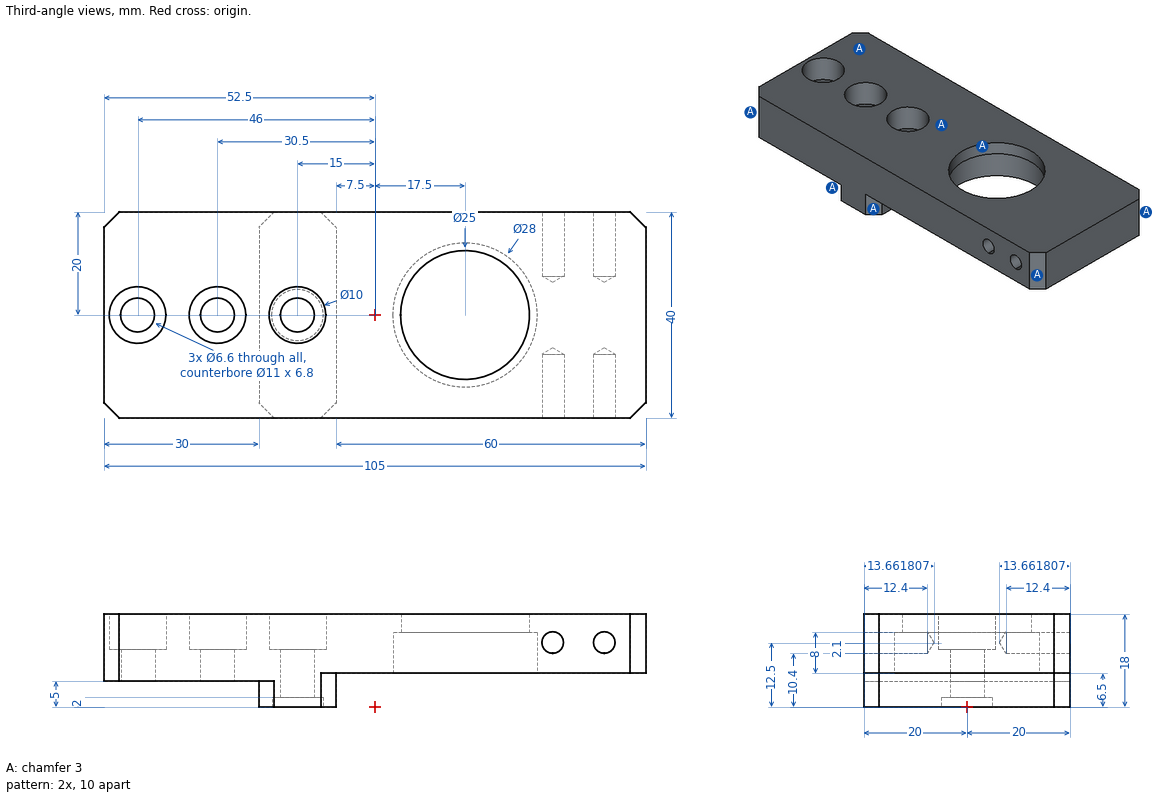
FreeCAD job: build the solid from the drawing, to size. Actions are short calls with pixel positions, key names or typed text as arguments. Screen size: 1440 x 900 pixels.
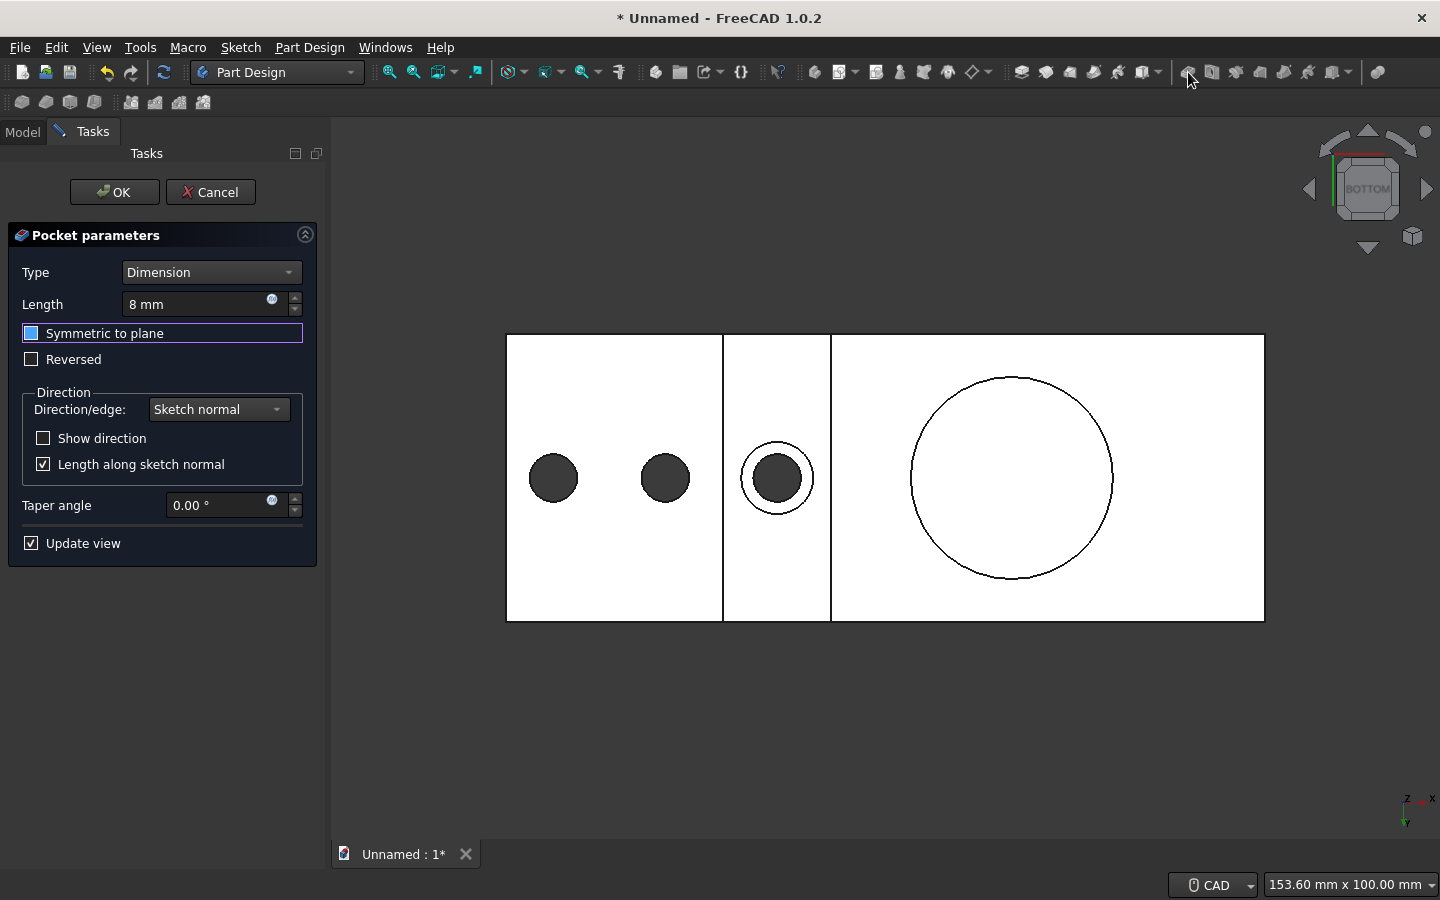
click(115, 192)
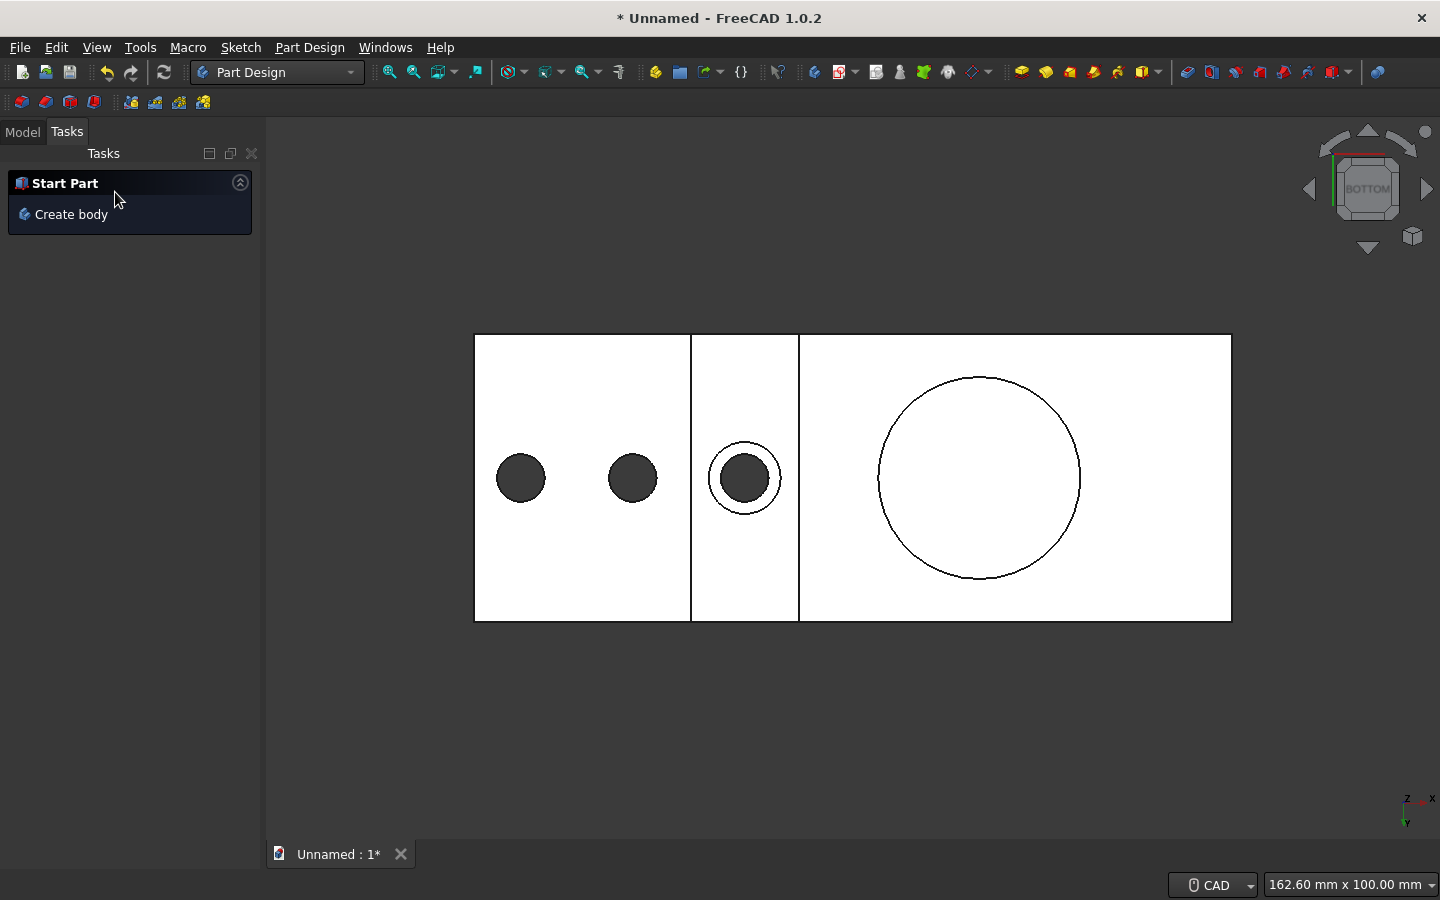
click(979, 477)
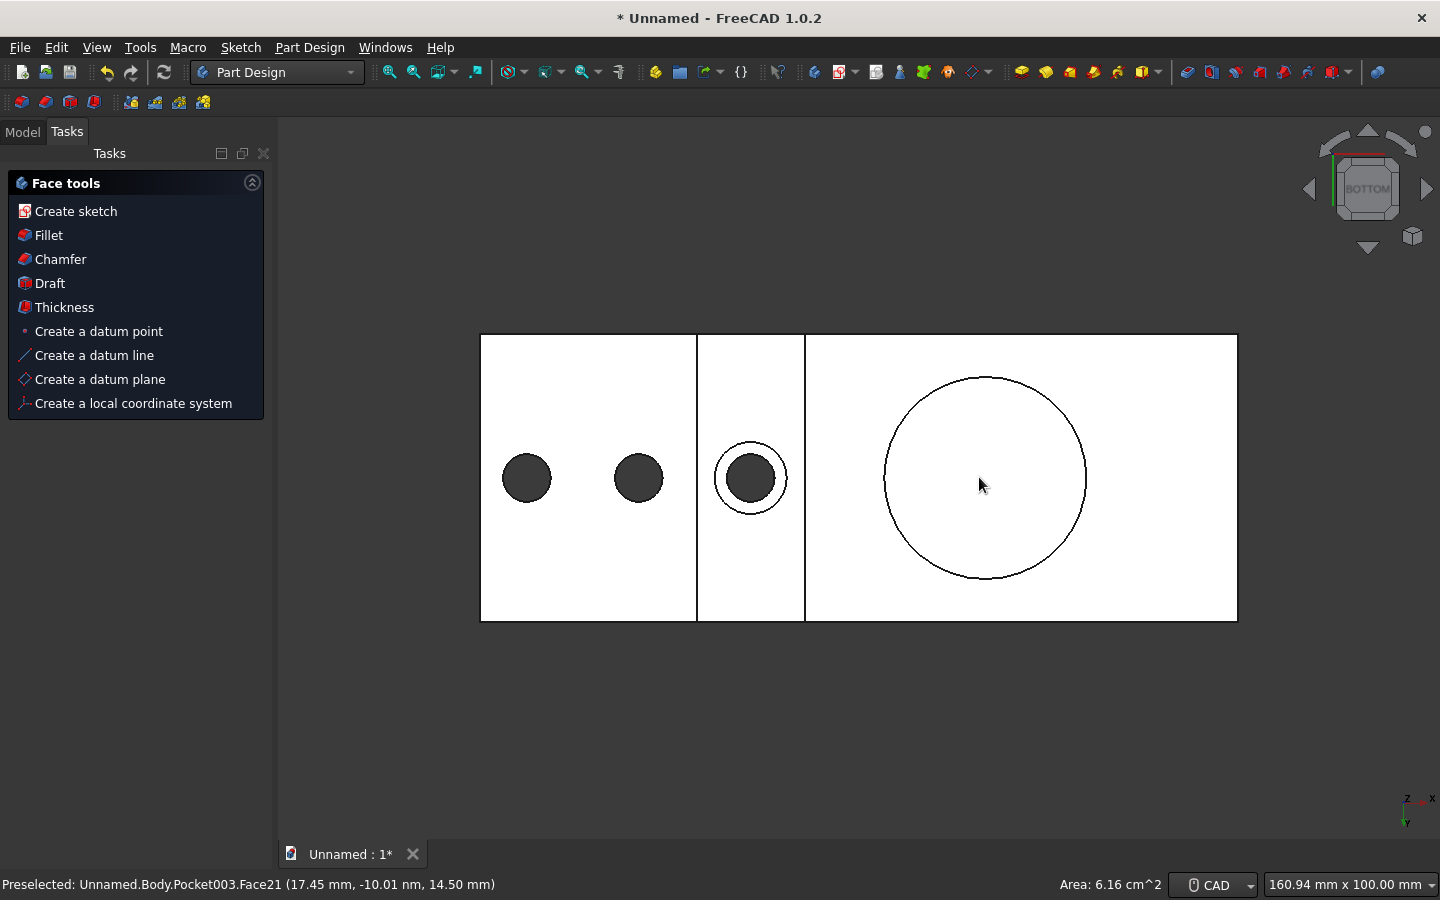
click(840, 72)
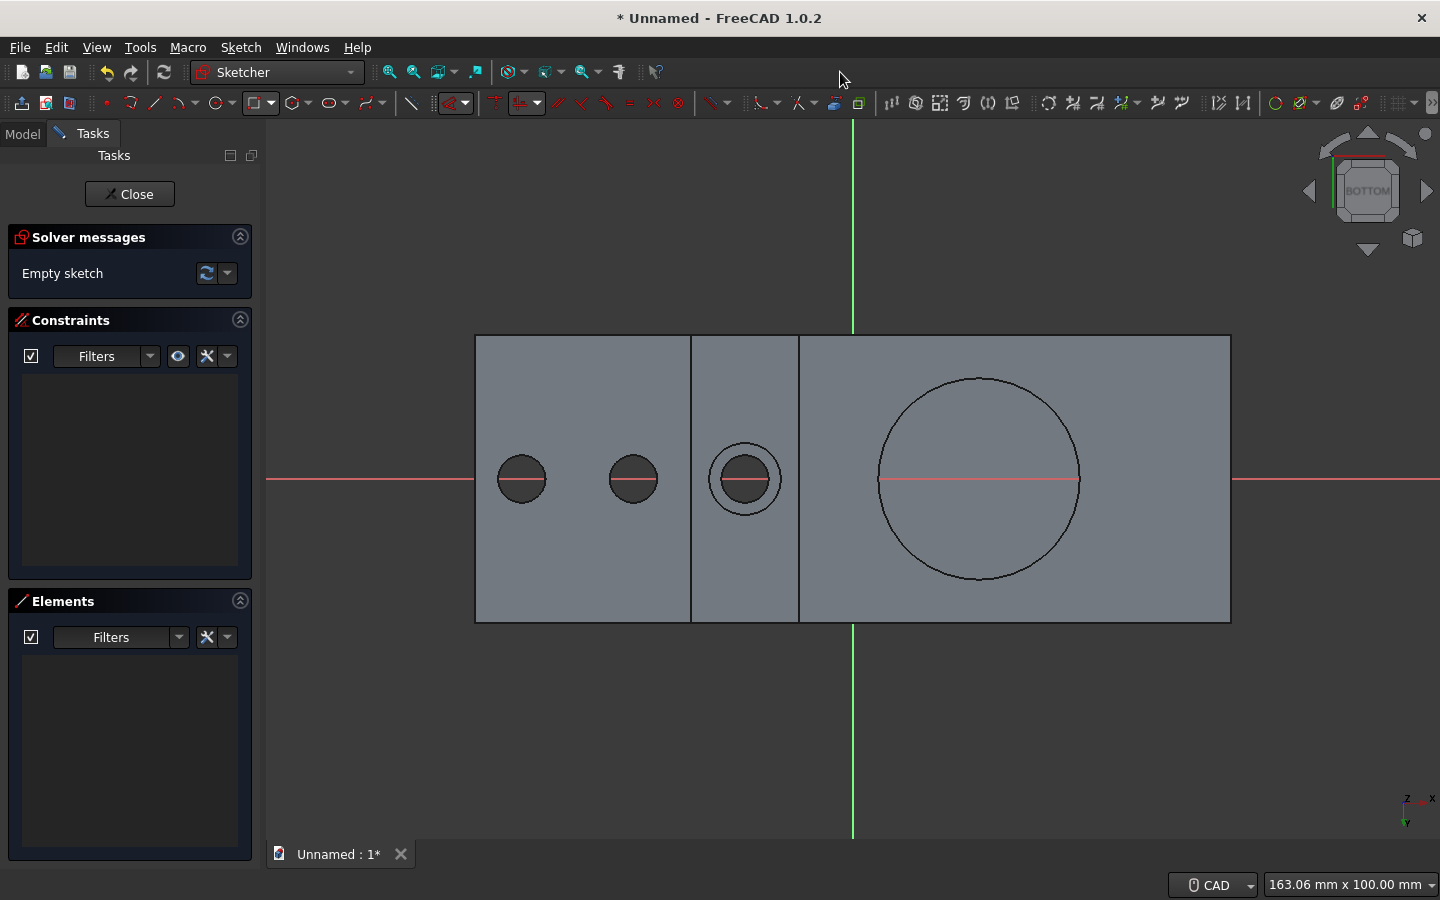
scroll(1064, 479, up, 5)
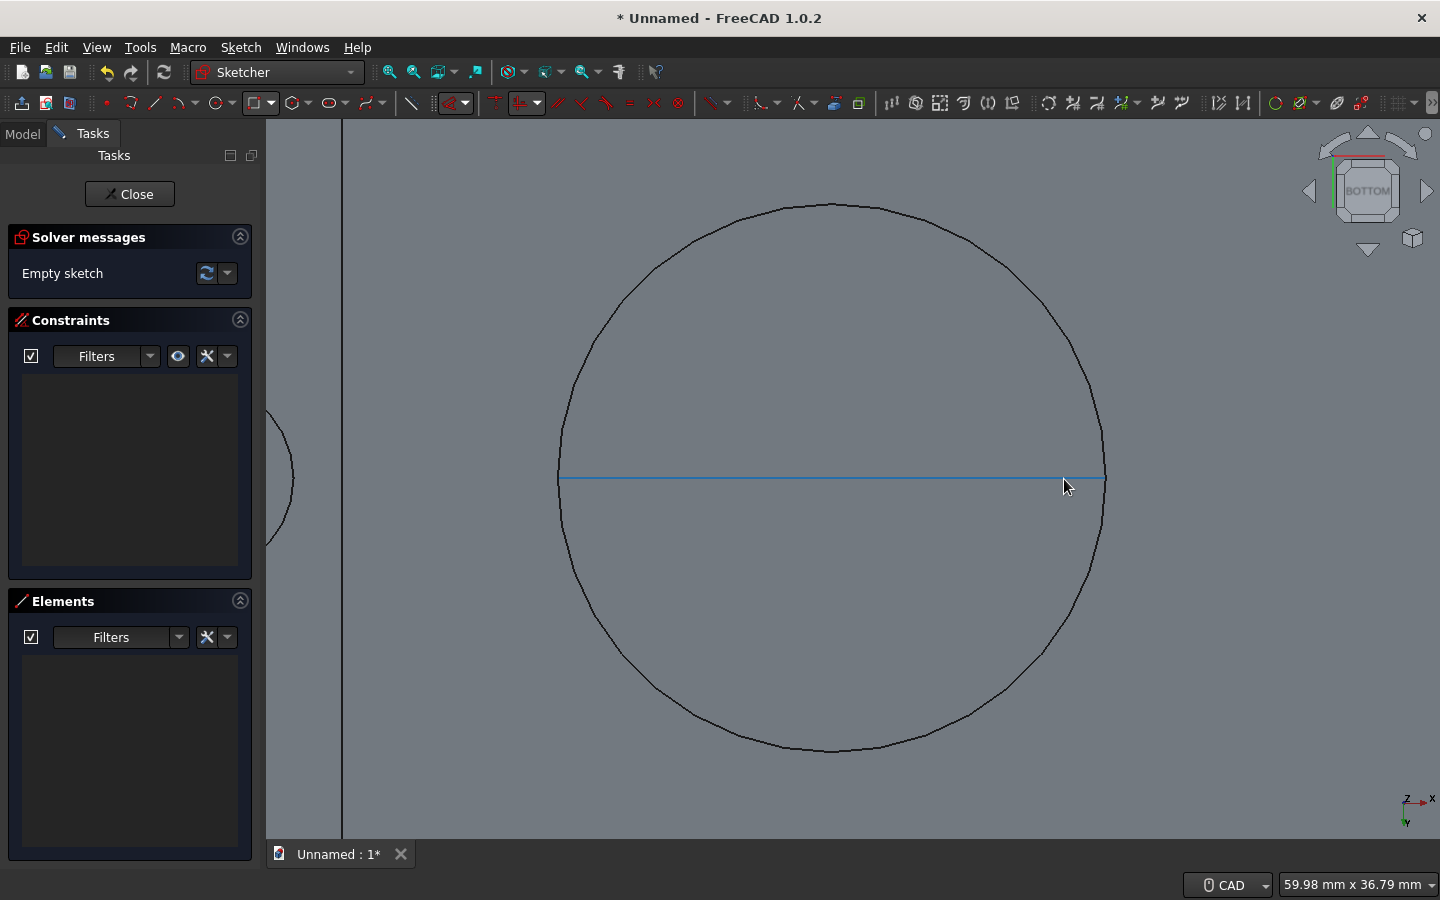
click(216, 104)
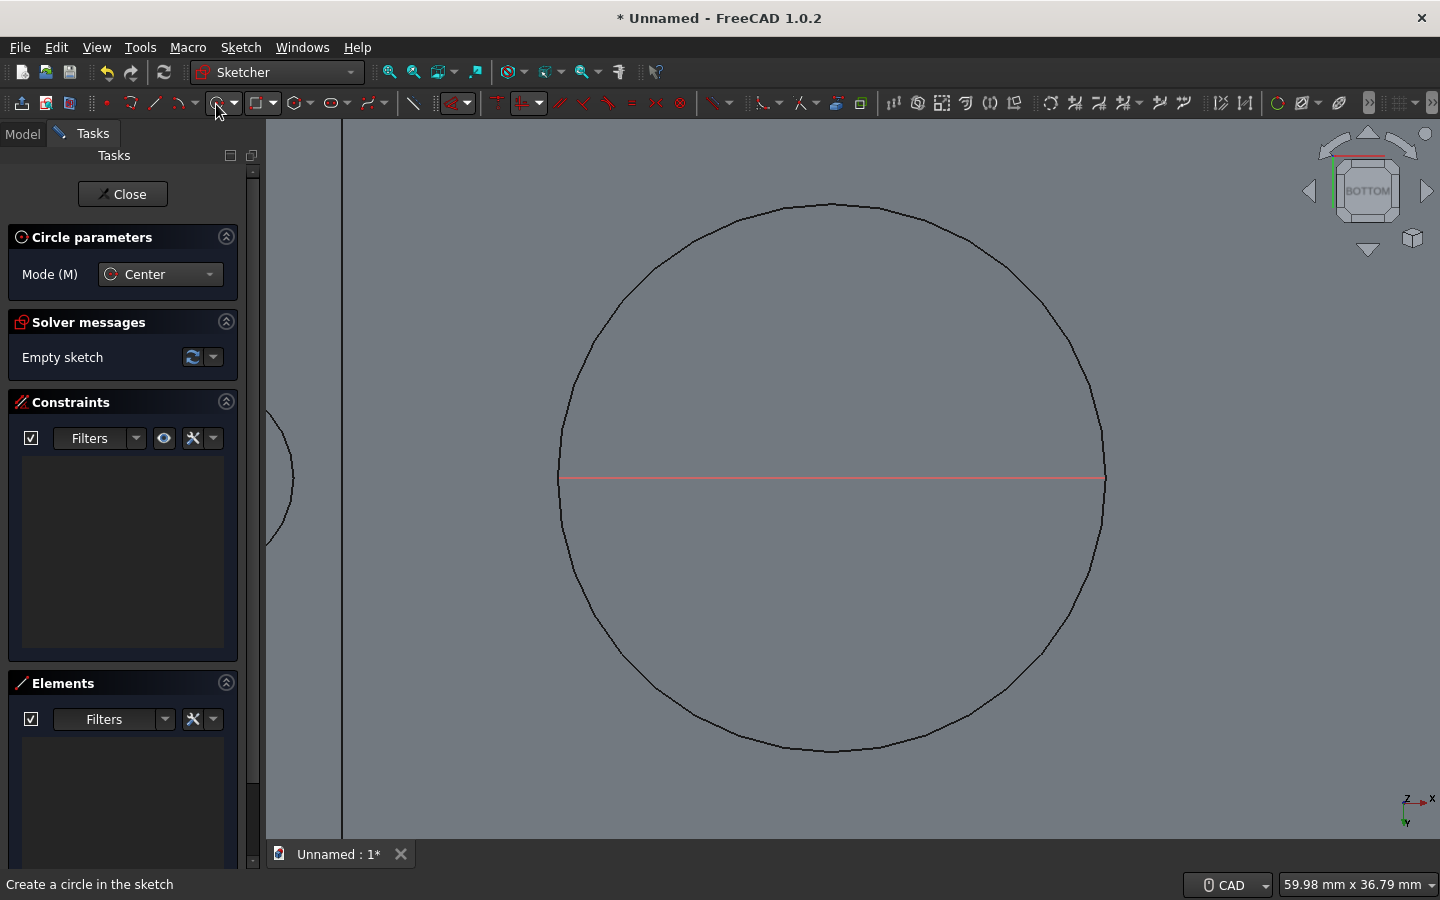
click(832, 478)
click(1005, 305)
key(Escape)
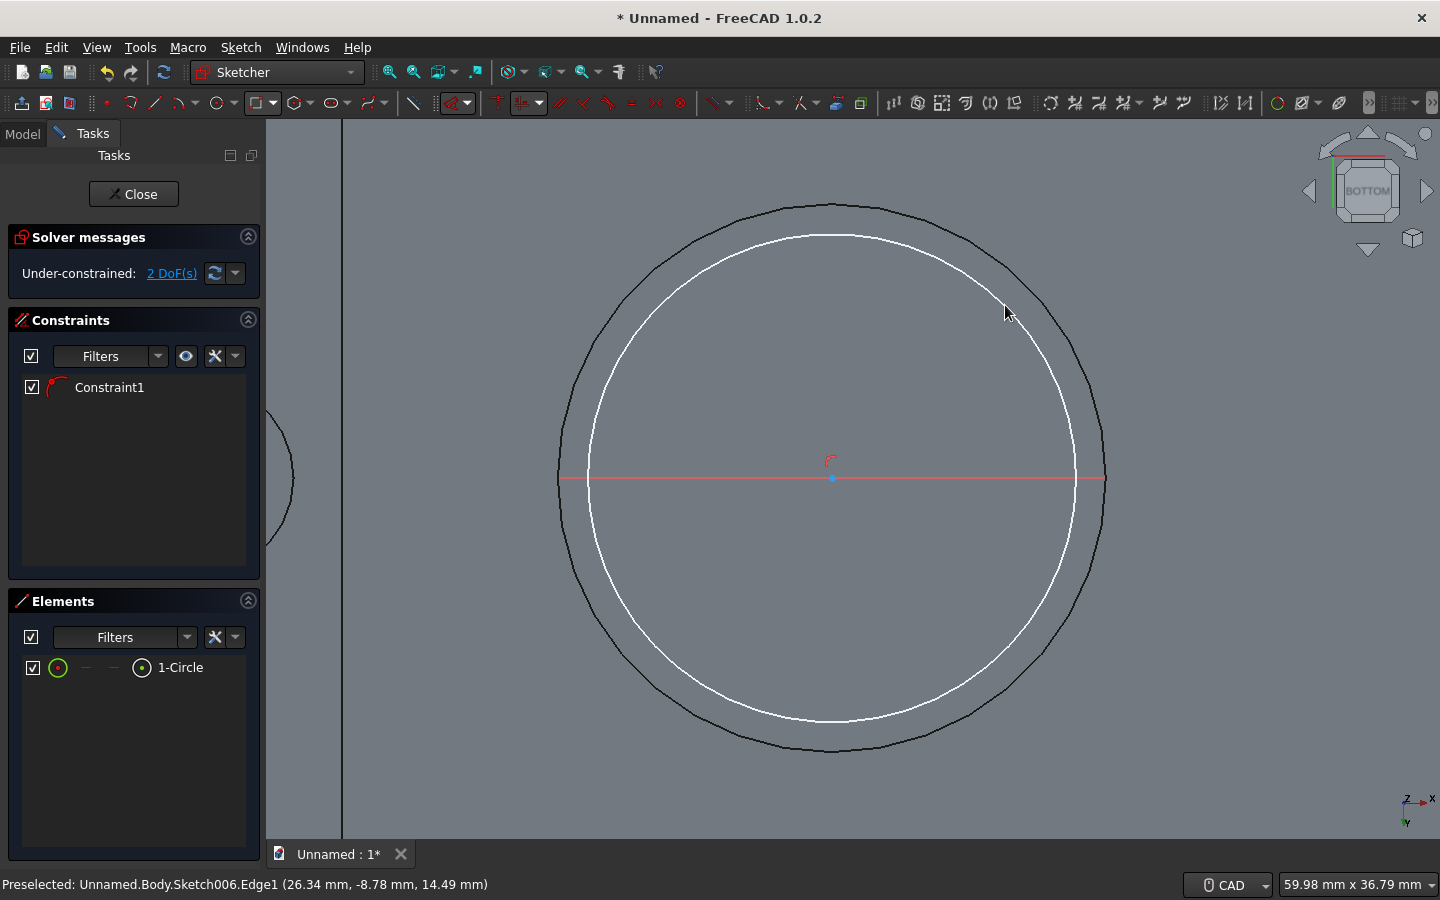
click(1004, 305)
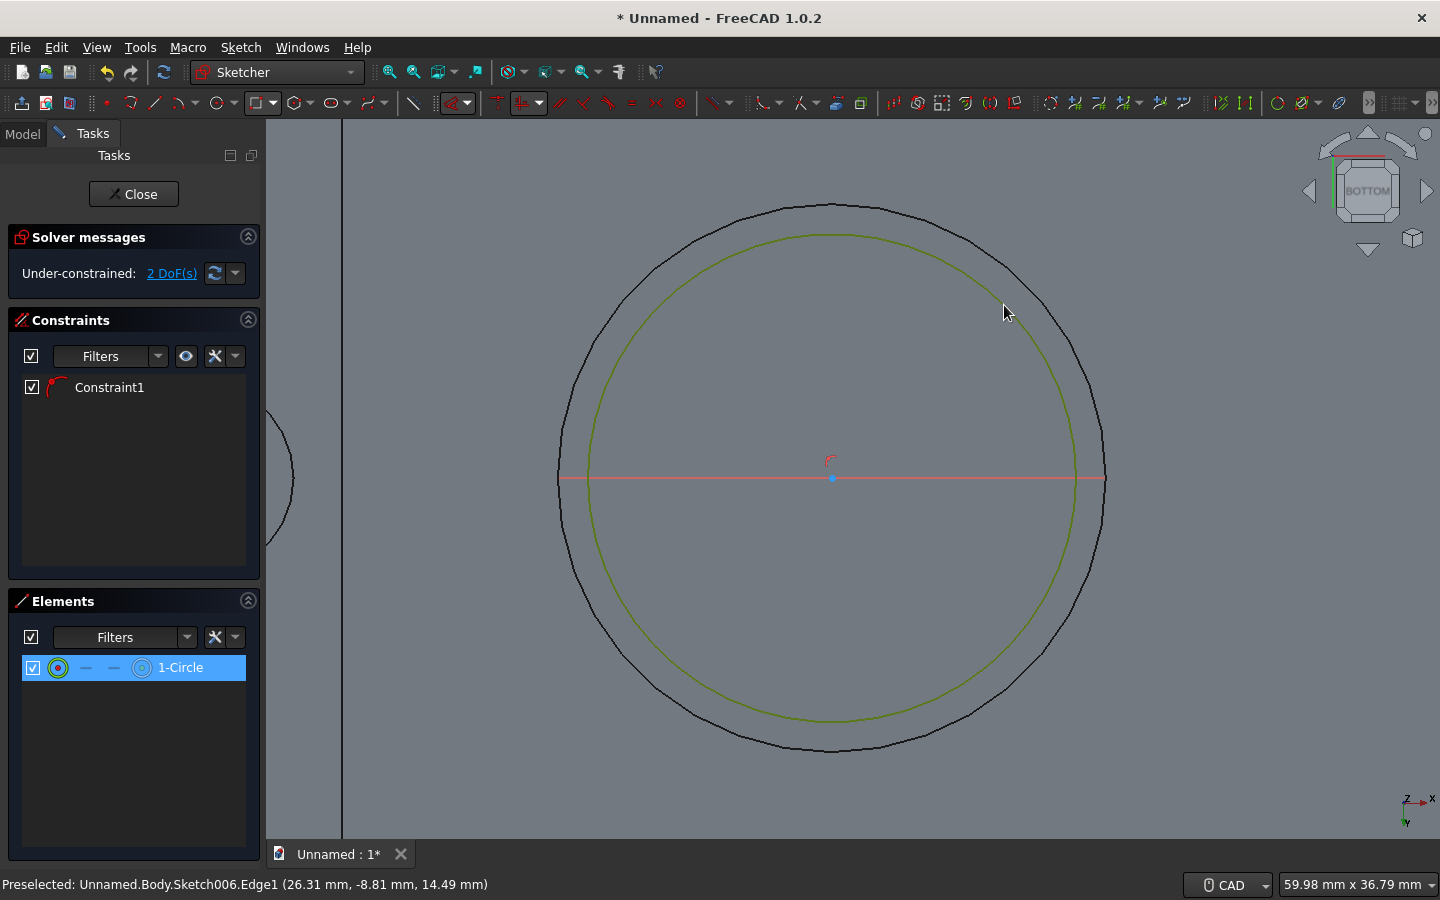
click(470, 104)